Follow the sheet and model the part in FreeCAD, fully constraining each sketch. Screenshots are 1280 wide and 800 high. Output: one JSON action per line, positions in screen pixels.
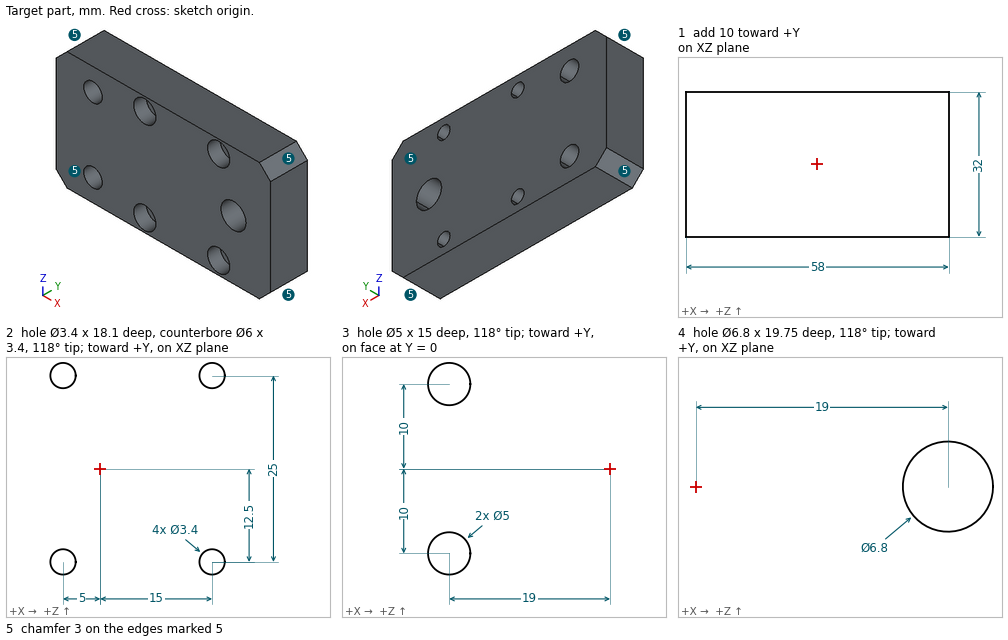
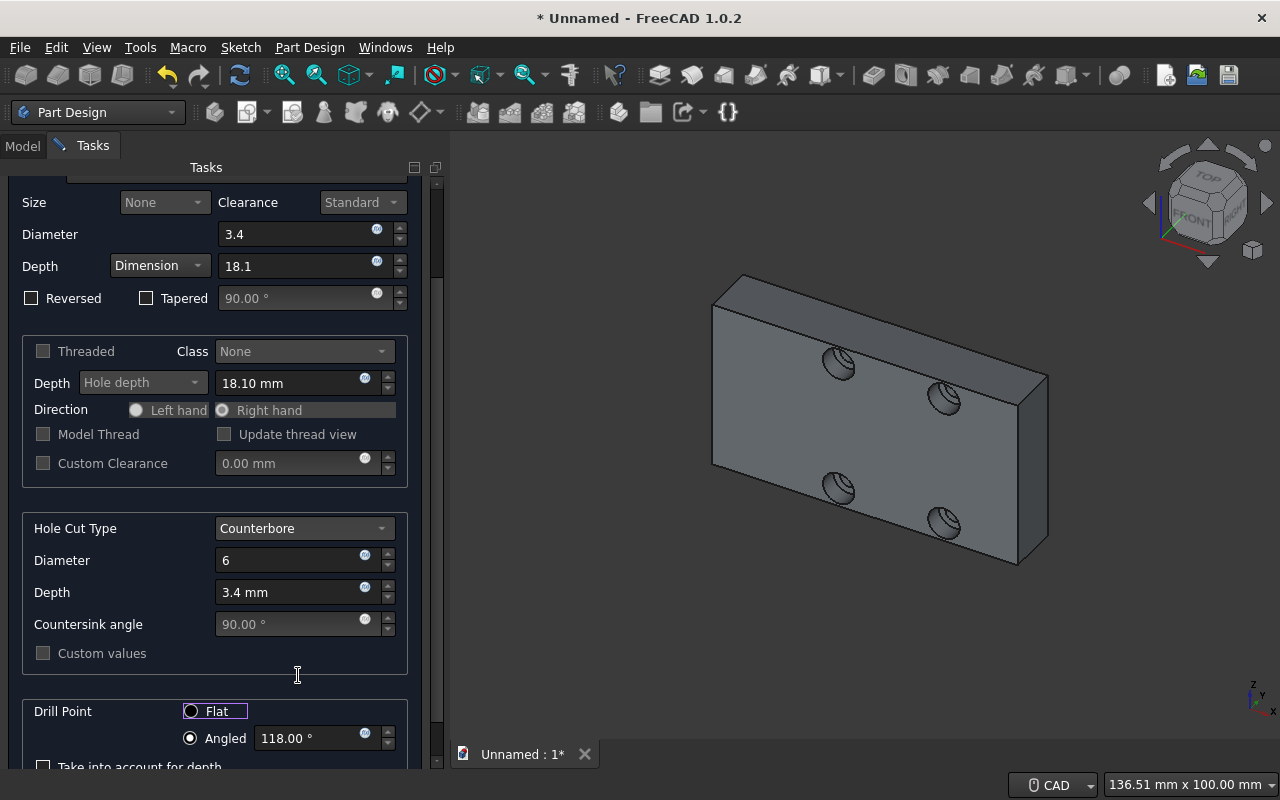
{"action": "scroll", "coordinate": [437, 472], "scroll_direction": "up", "scroll_amount": 3}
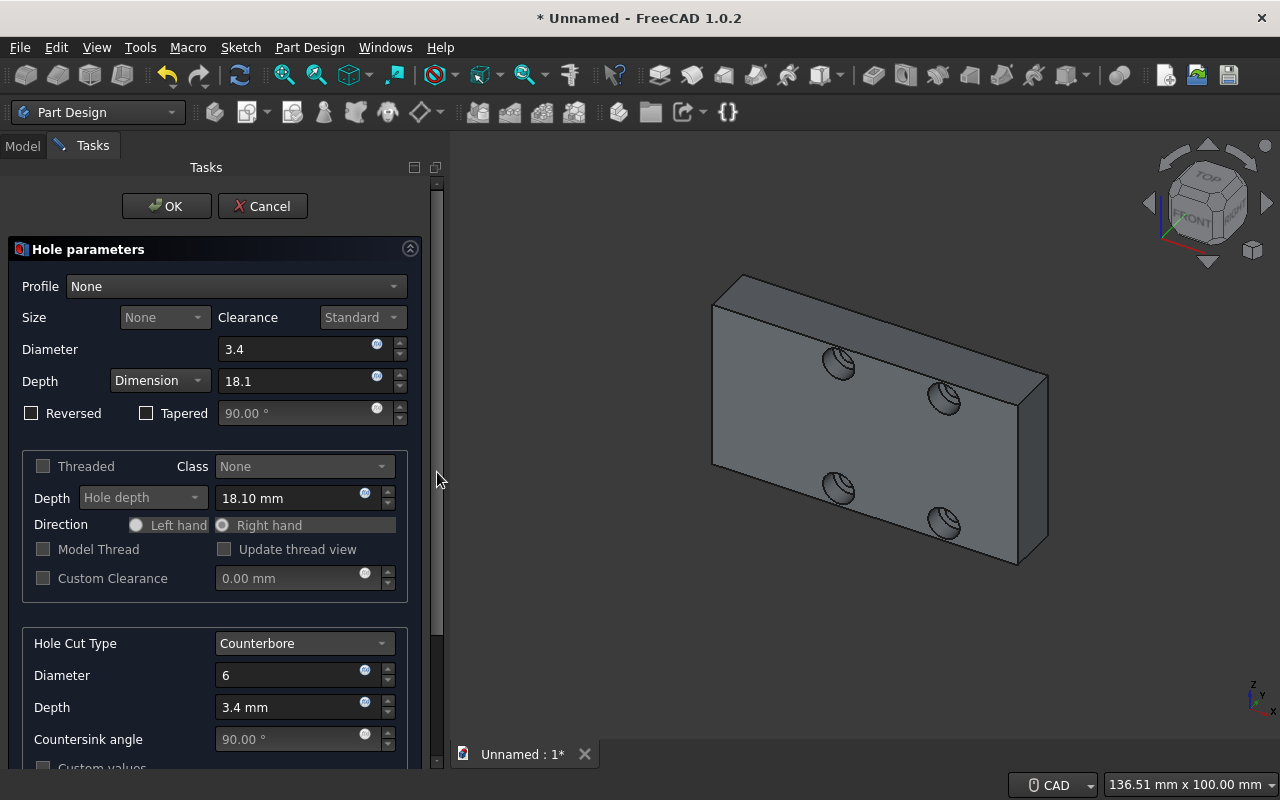
{"action": "left_click", "coordinate": [167, 206]}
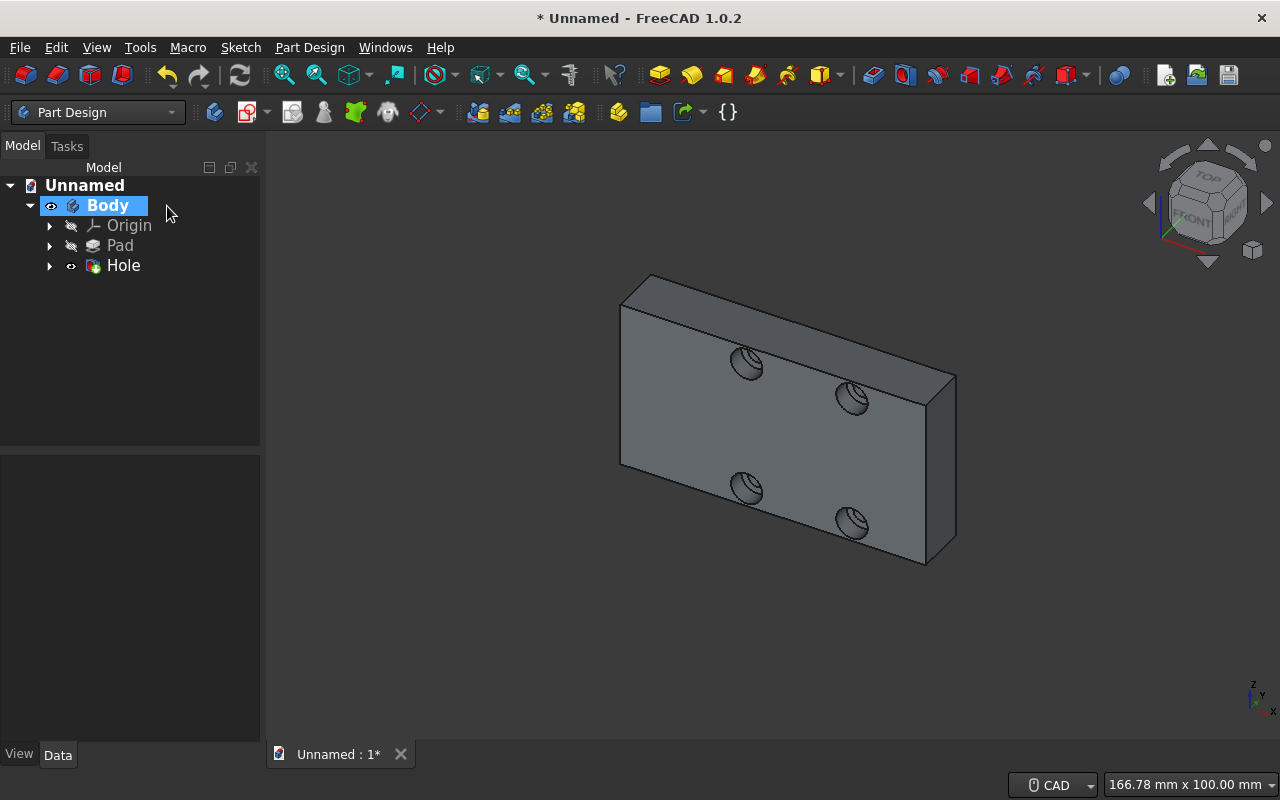
{"action": "left_click", "coordinate": [686, 405]}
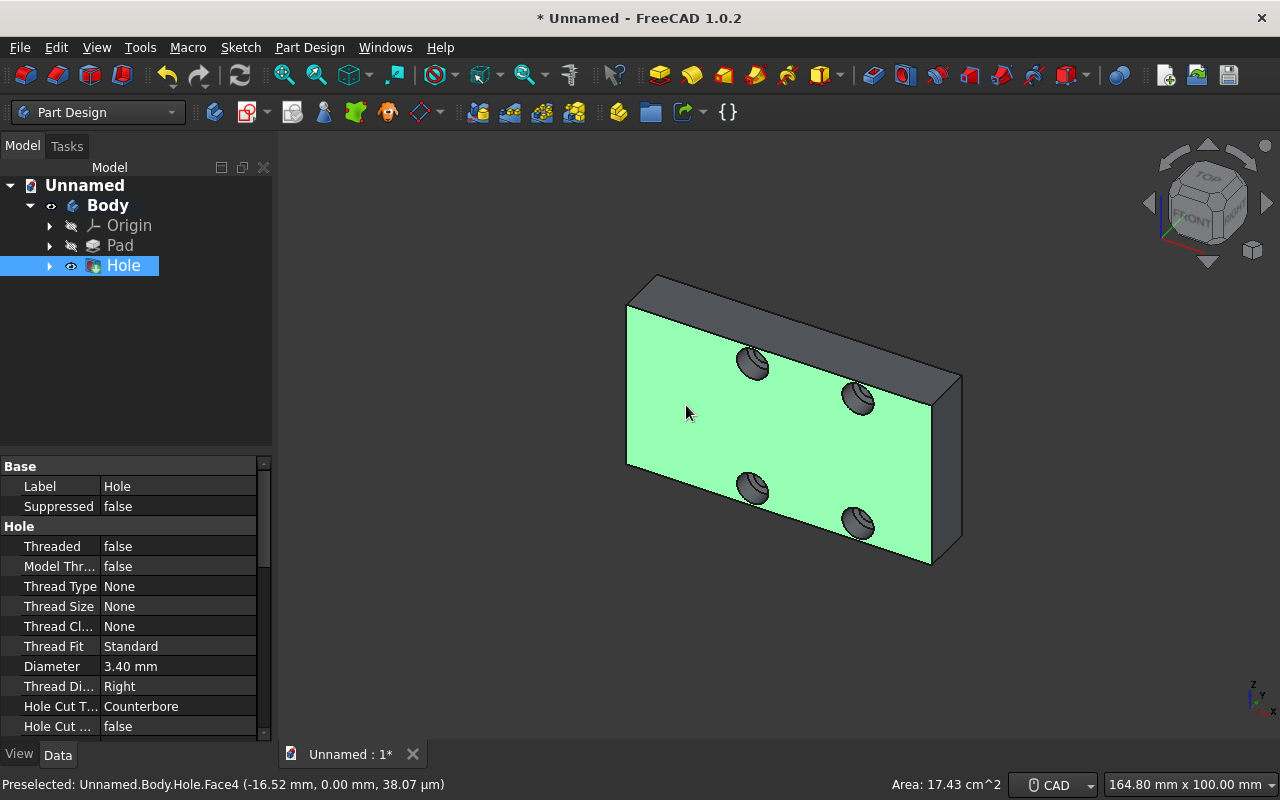
{"action": "left_click", "coordinate": [248, 112]}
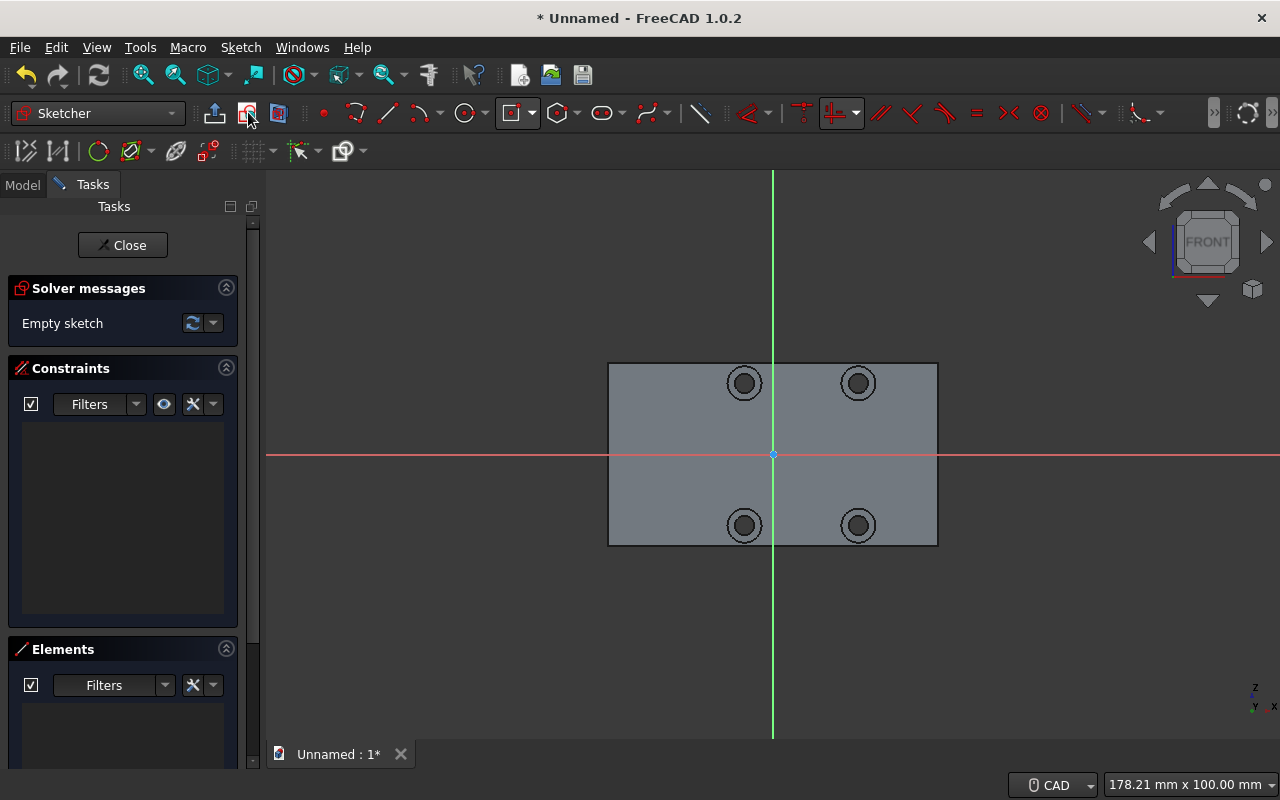
{"action": "scroll", "coordinate": [716, 454], "scroll_direction": "up", "scroll_amount": 5}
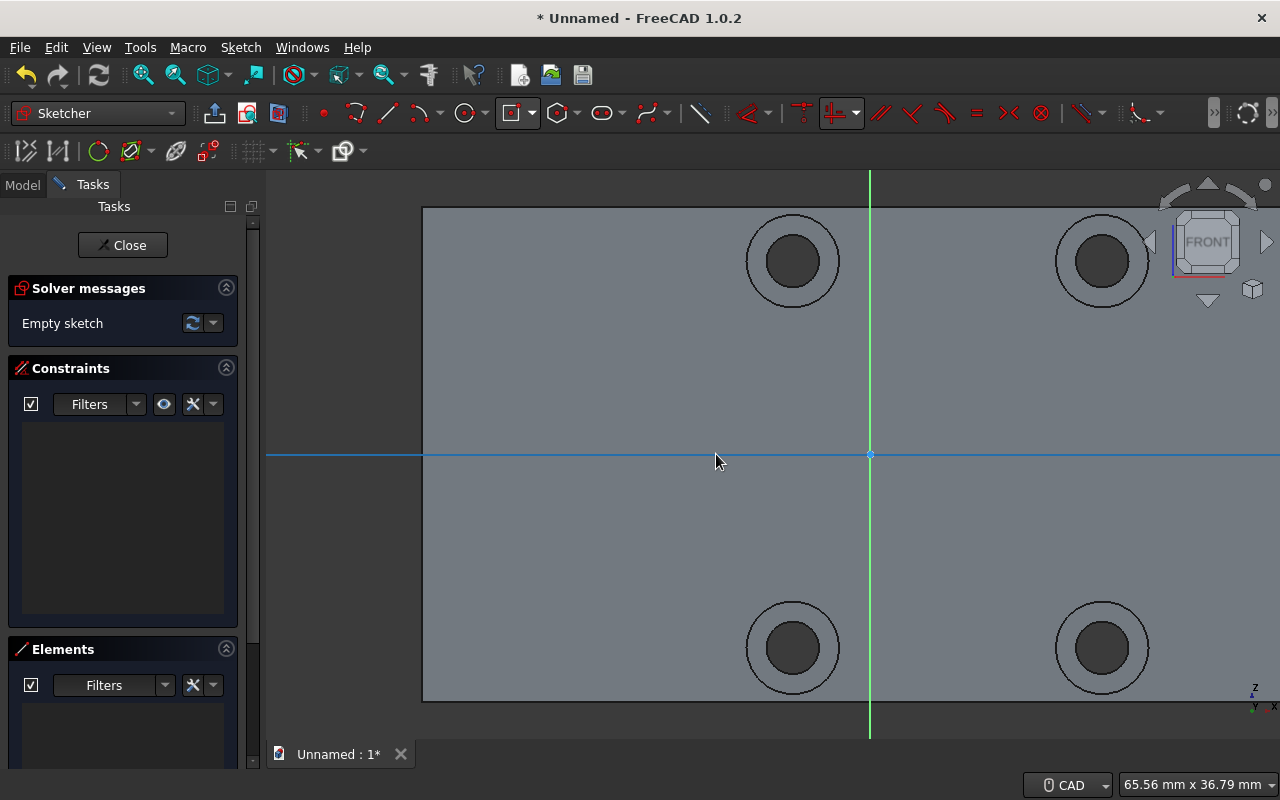
{"action": "left_click", "coordinate": [466, 114]}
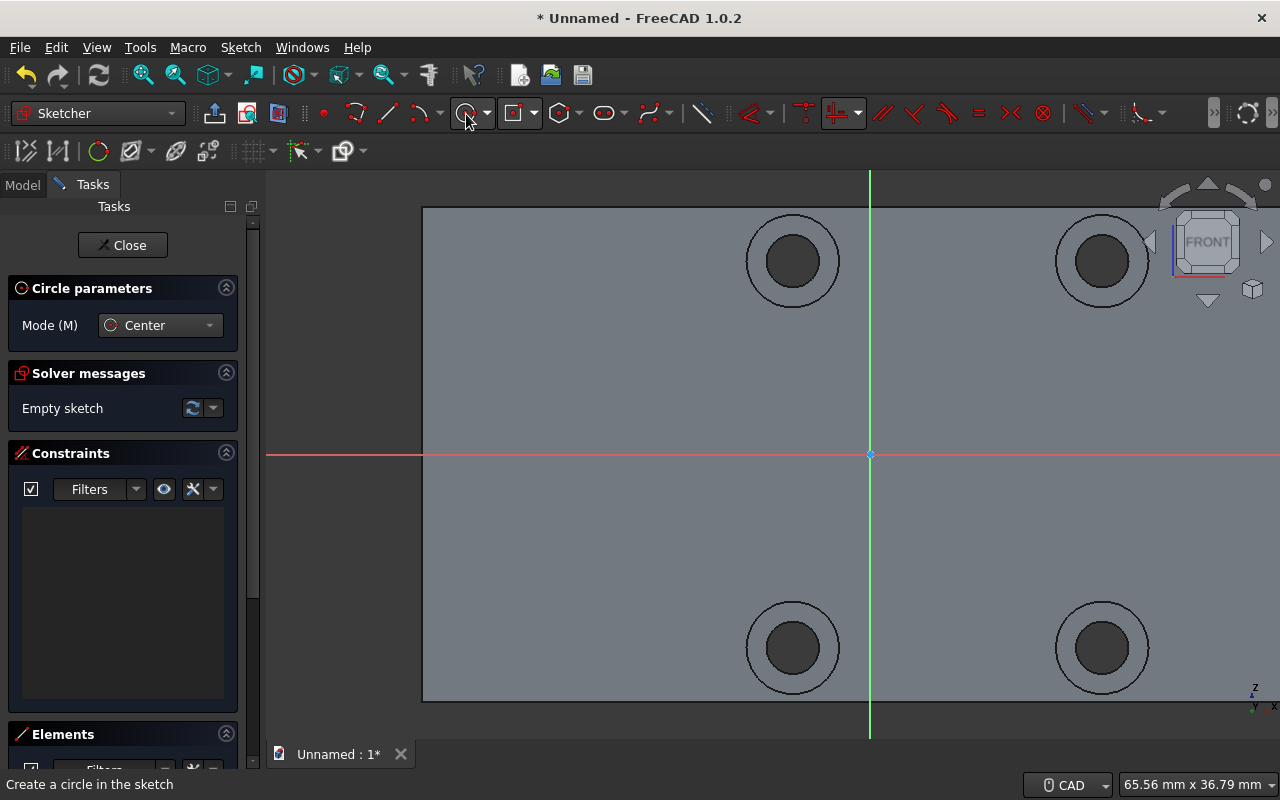
{"action": "left_click", "coordinate": [576, 609]}
{"action": "left_click", "coordinate": [604, 582]}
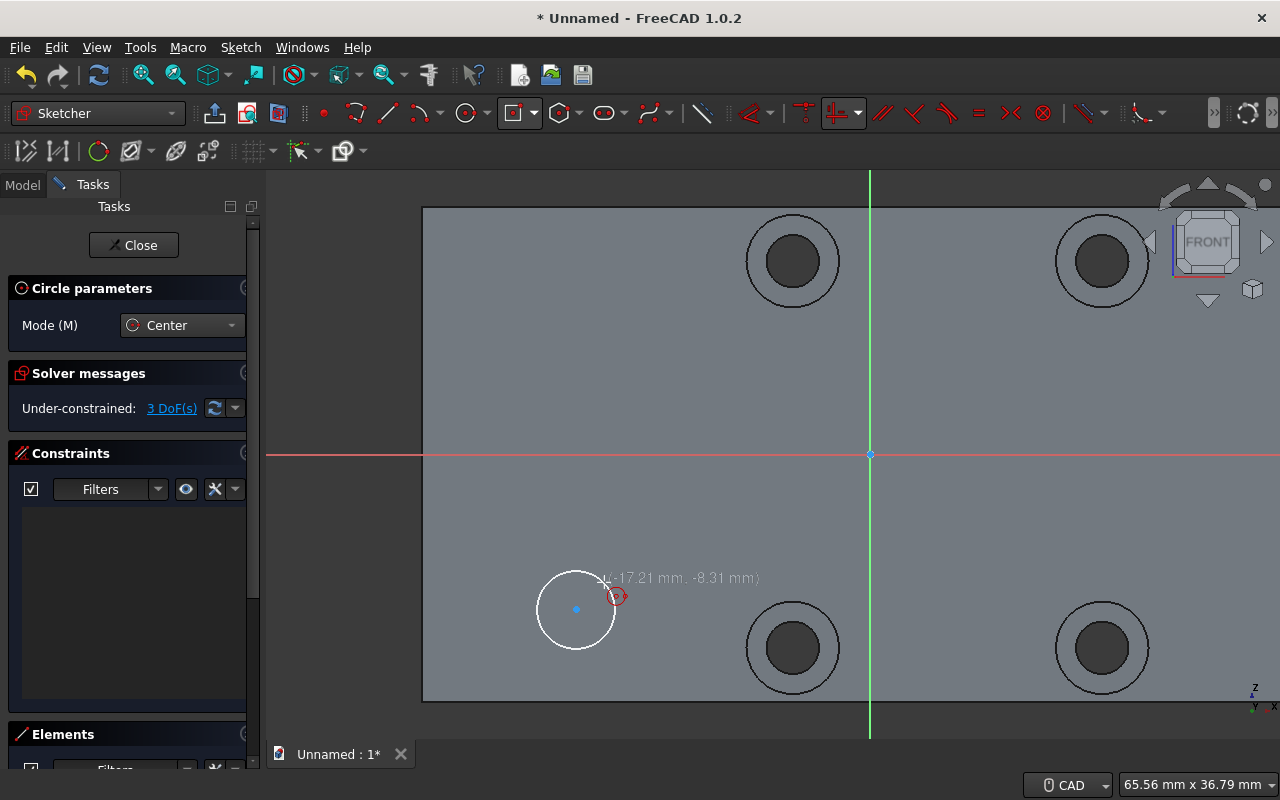
{"action": "left_click", "coordinate": [576, 300]}
{"action": "left_click", "coordinate": [604, 272]}
{"action": "key", "text": "Escape"}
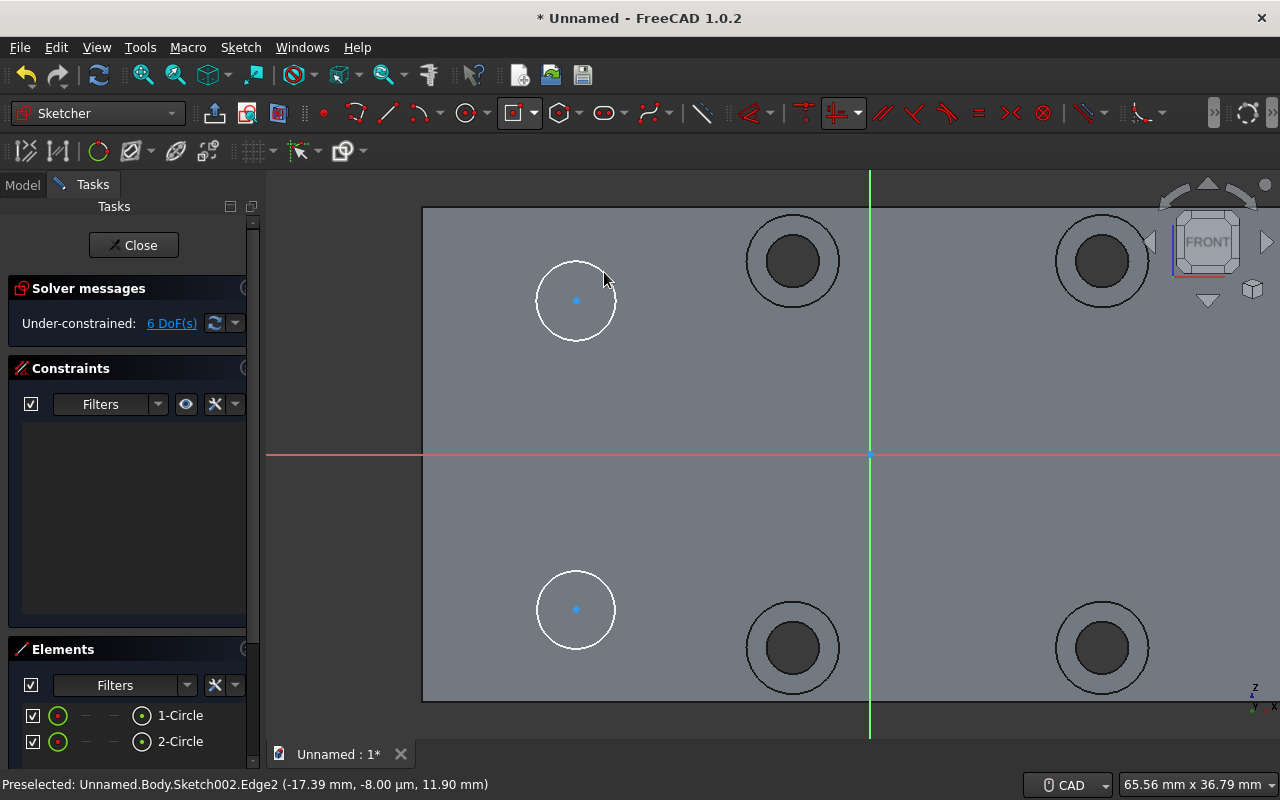
{"action": "left_click", "coordinate": [603, 582]}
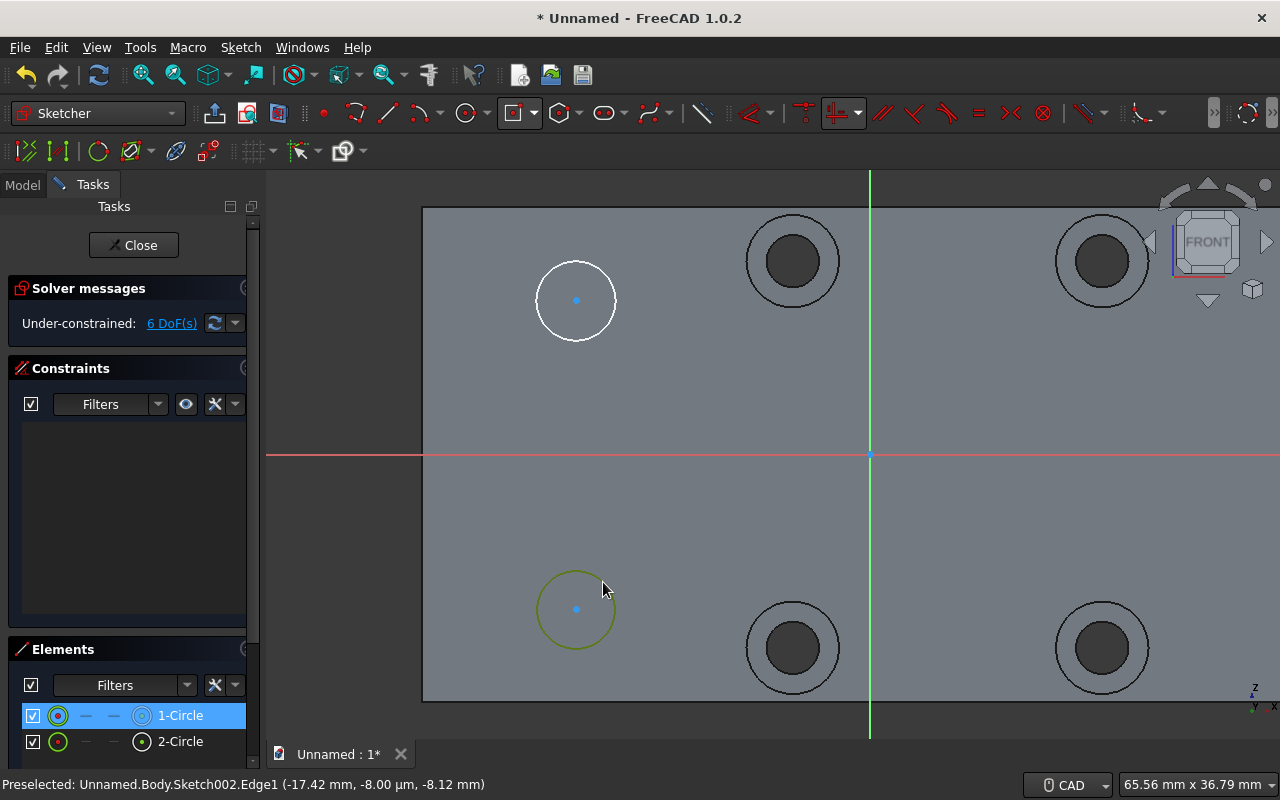
{"action": "left_click", "coordinate": [604, 273]}